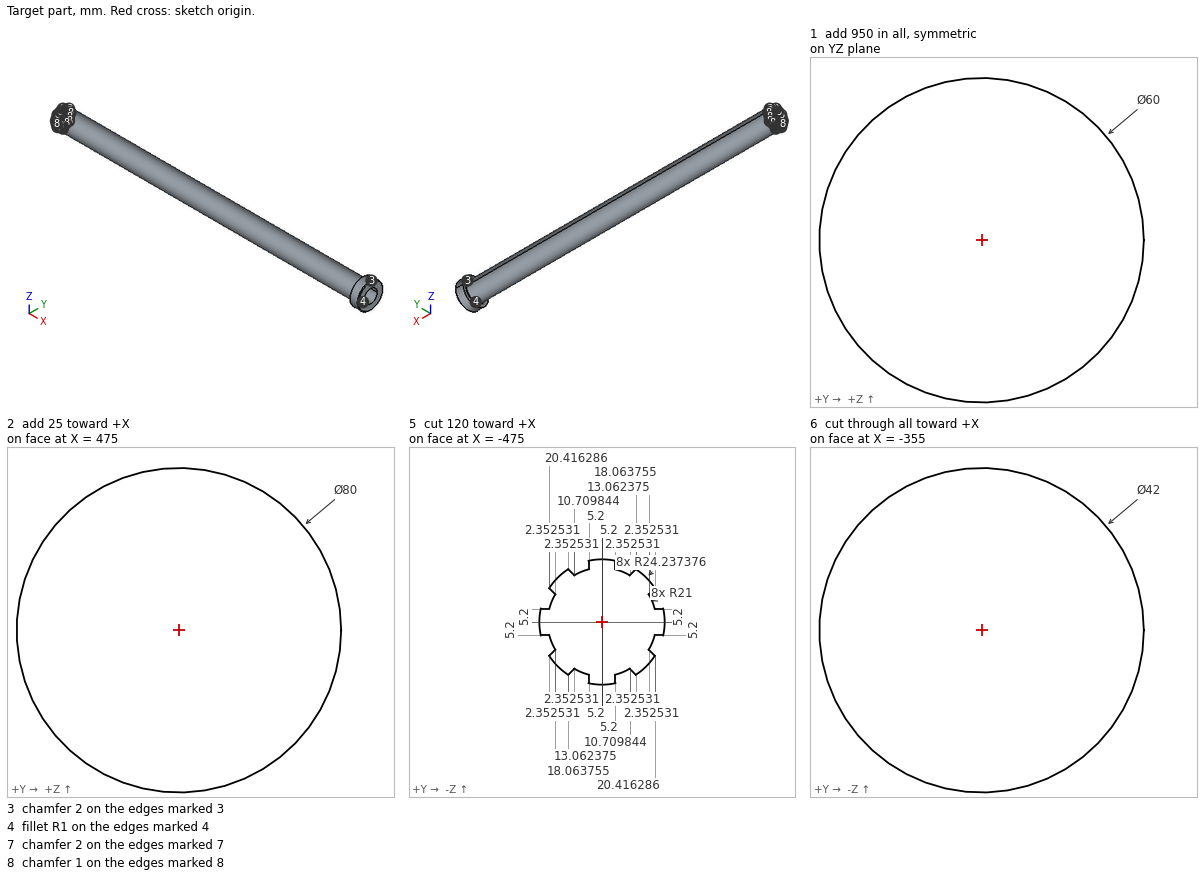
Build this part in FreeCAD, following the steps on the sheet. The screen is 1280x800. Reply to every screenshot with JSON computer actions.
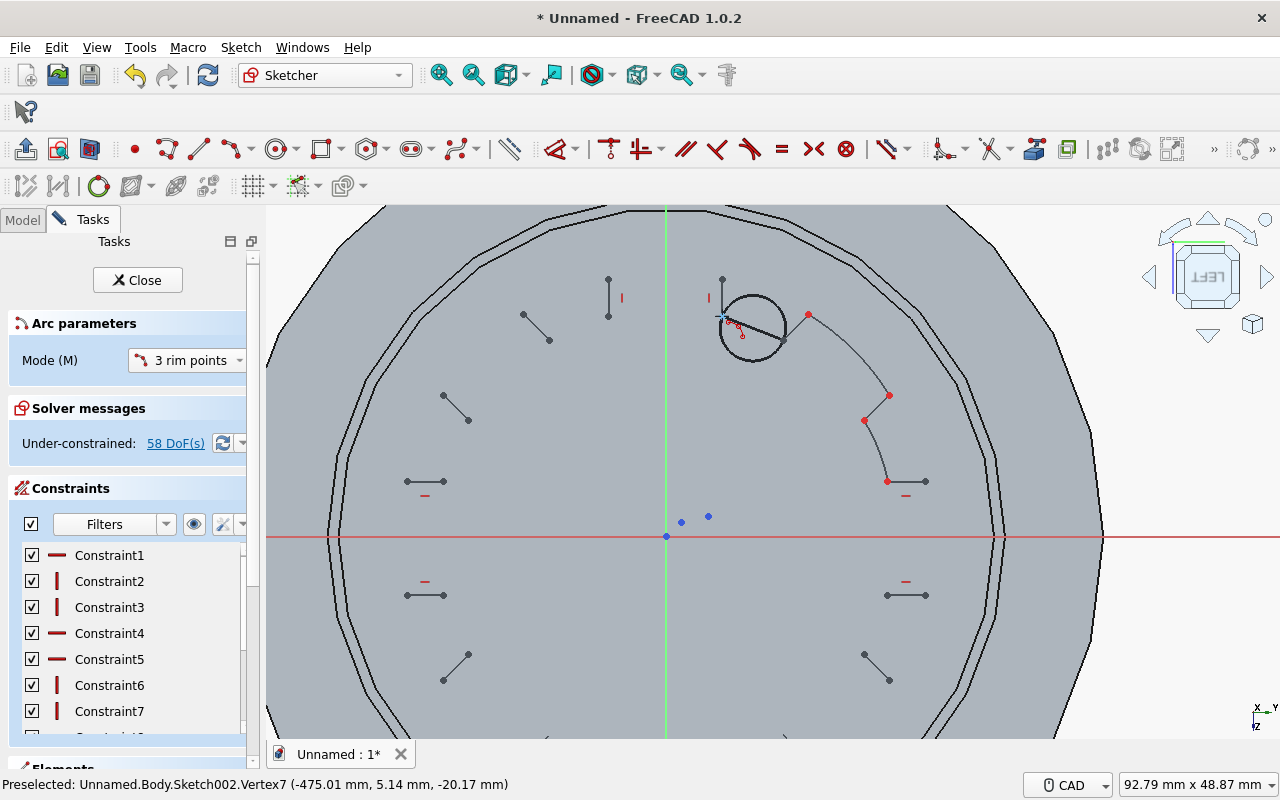
{"action": "scroll", "coordinate": [754, 325], "scroll_direction": "up", "scroll_amount": 10}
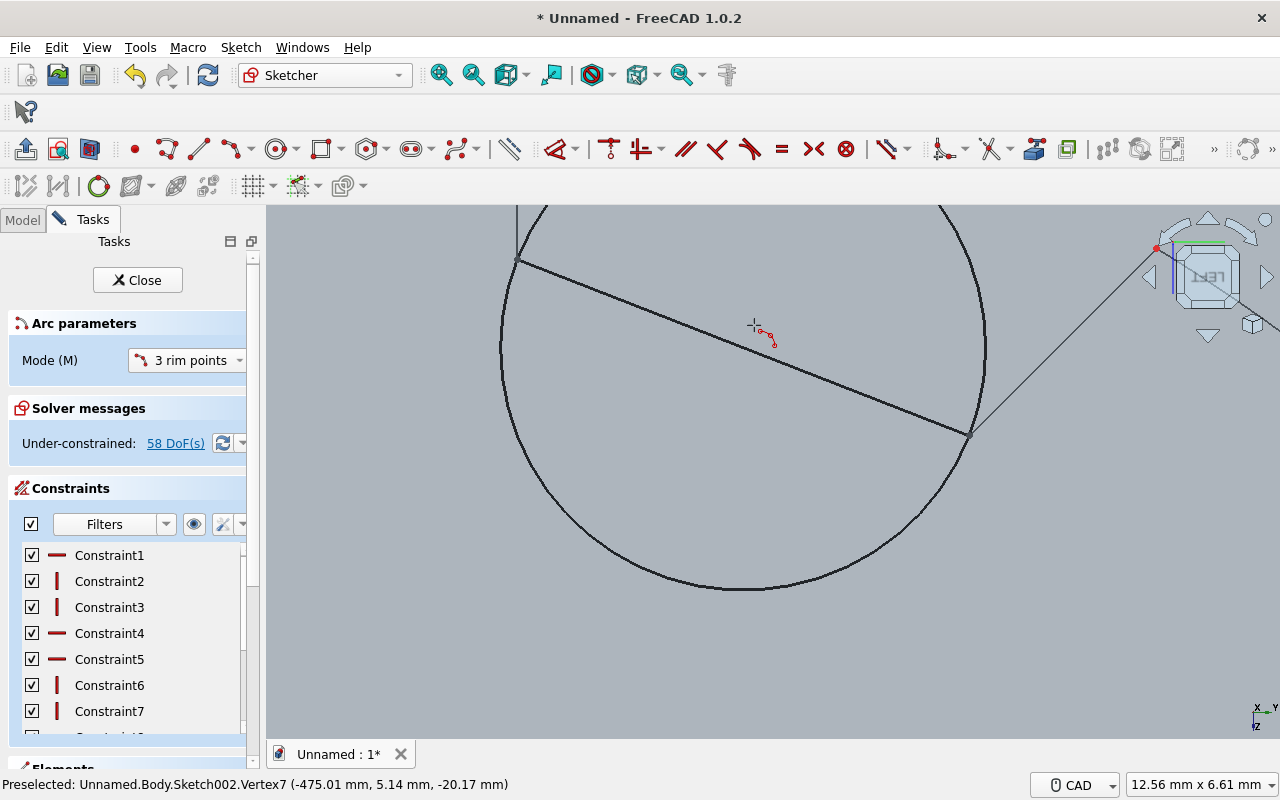
{"action": "left_click", "coordinate": [751, 322]}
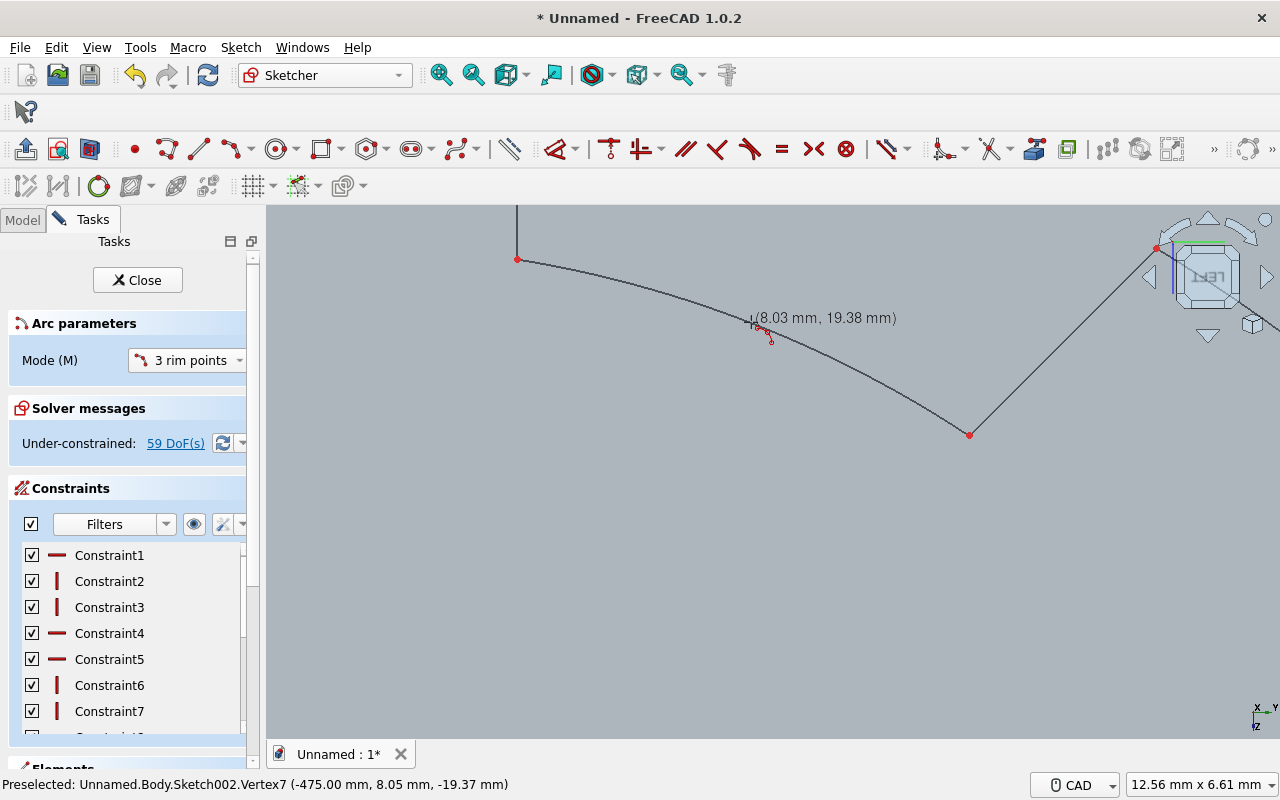
{"action": "scroll", "coordinate": [765, 331], "scroll_direction": "down", "scroll_amount": 12}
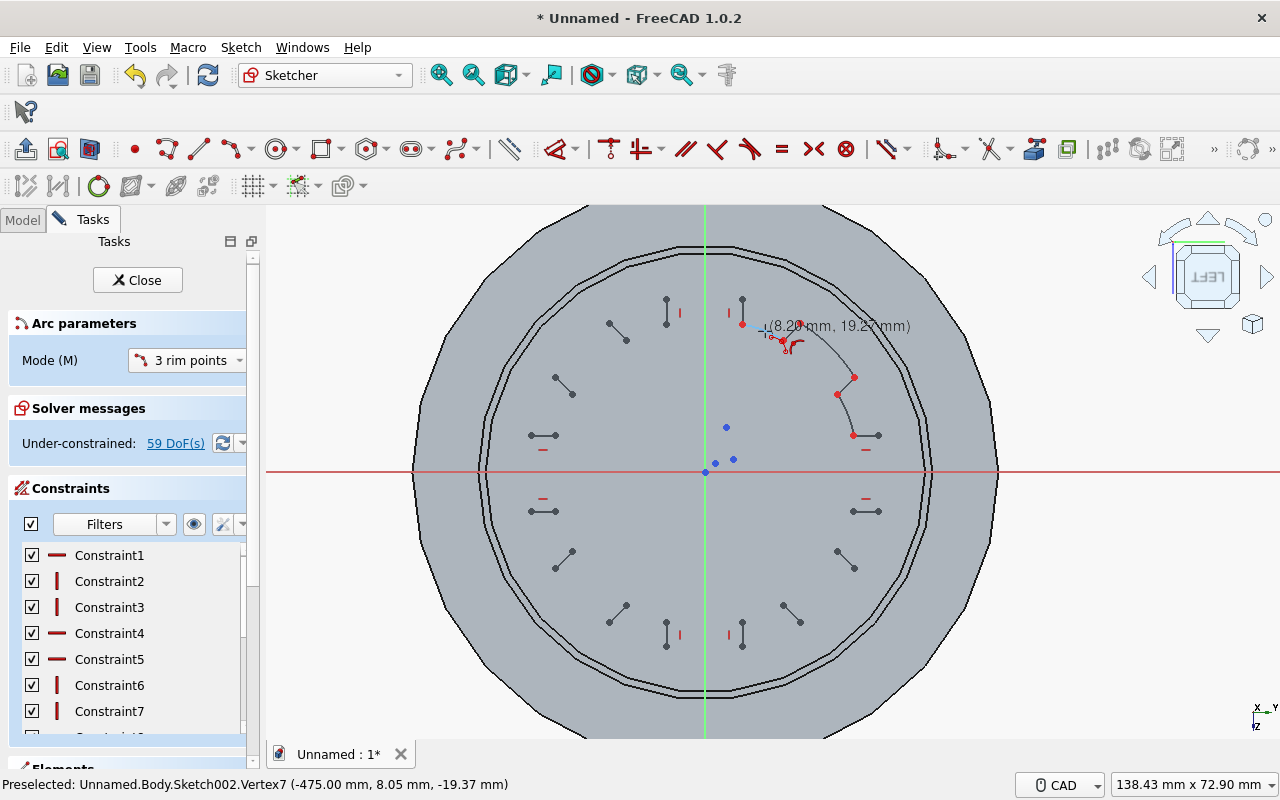
{"action": "scroll", "coordinate": [743, 299], "scroll_direction": "up", "scroll_amount": 2}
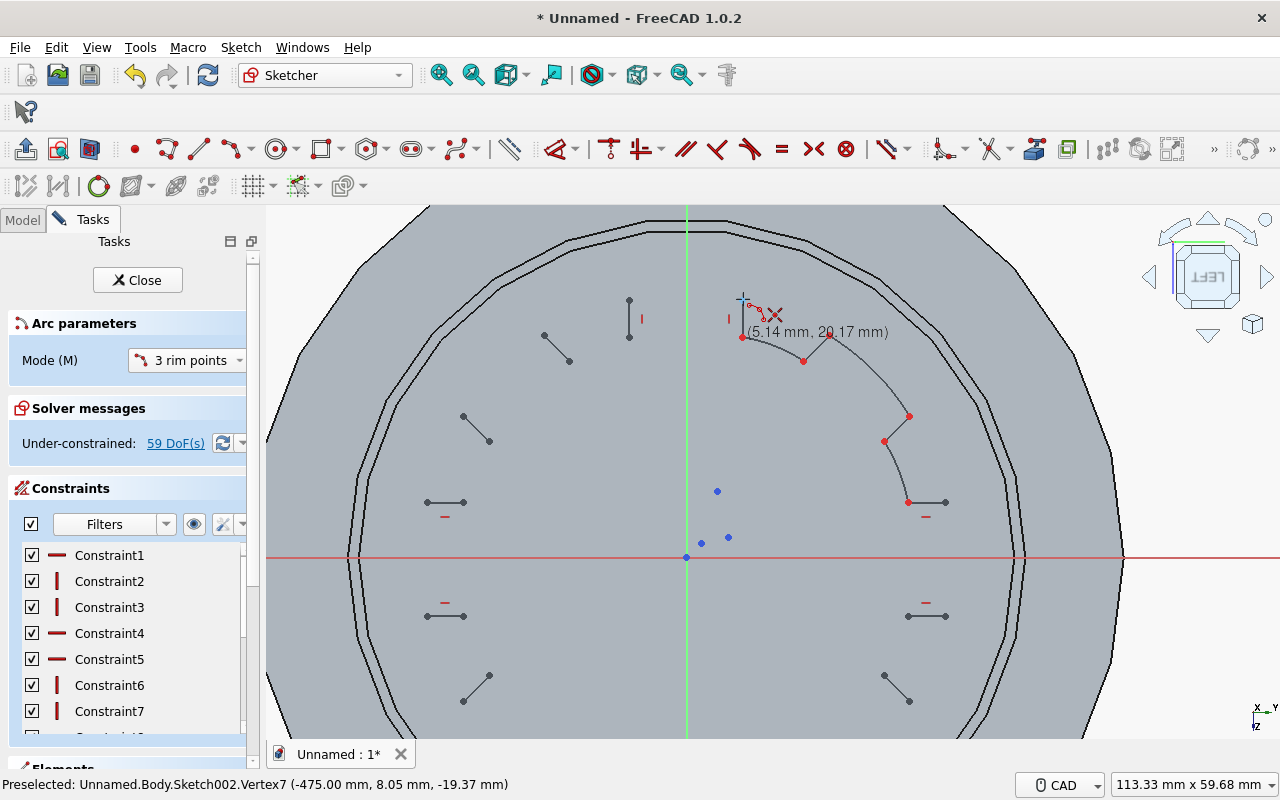
{"action": "left_click", "coordinate": [743, 300]}
{"action": "left_click", "coordinate": [629, 300]}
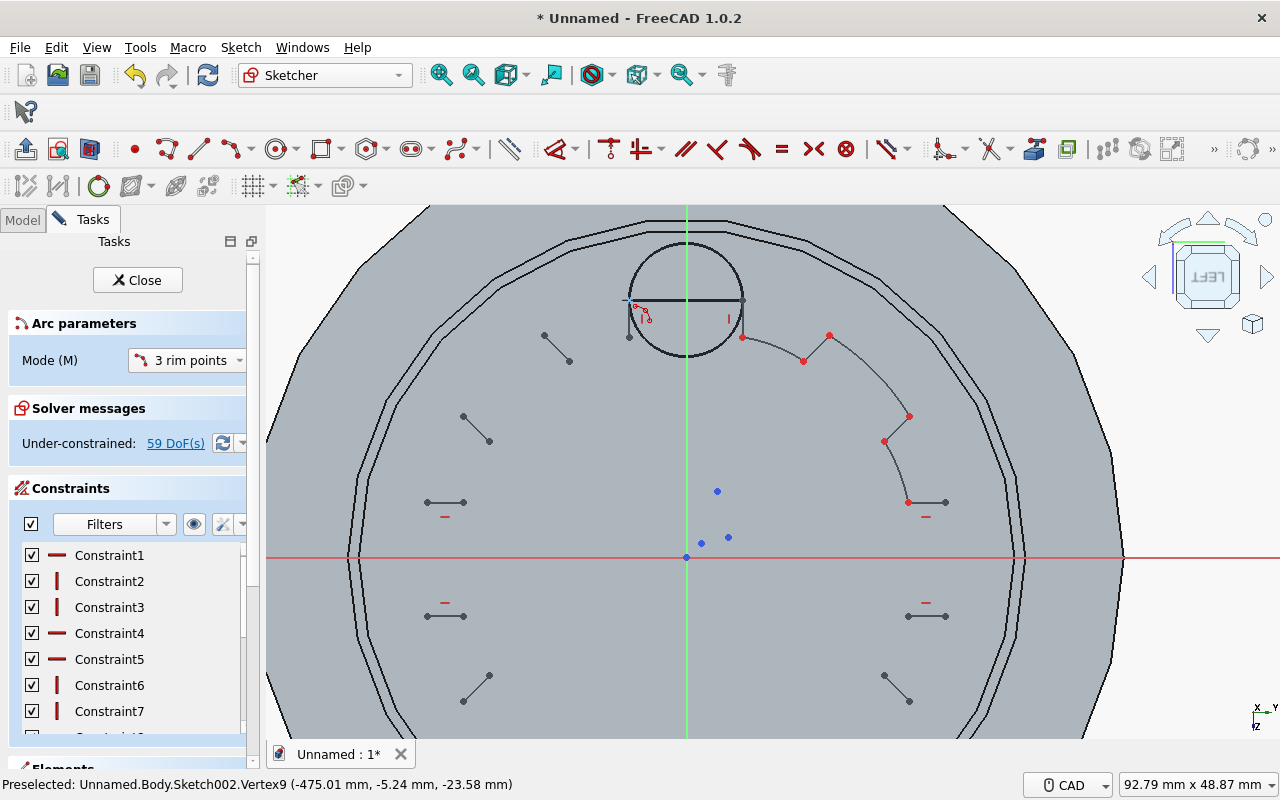
{"action": "scroll", "coordinate": [698, 293], "scroll_direction": "up", "scroll_amount": 5}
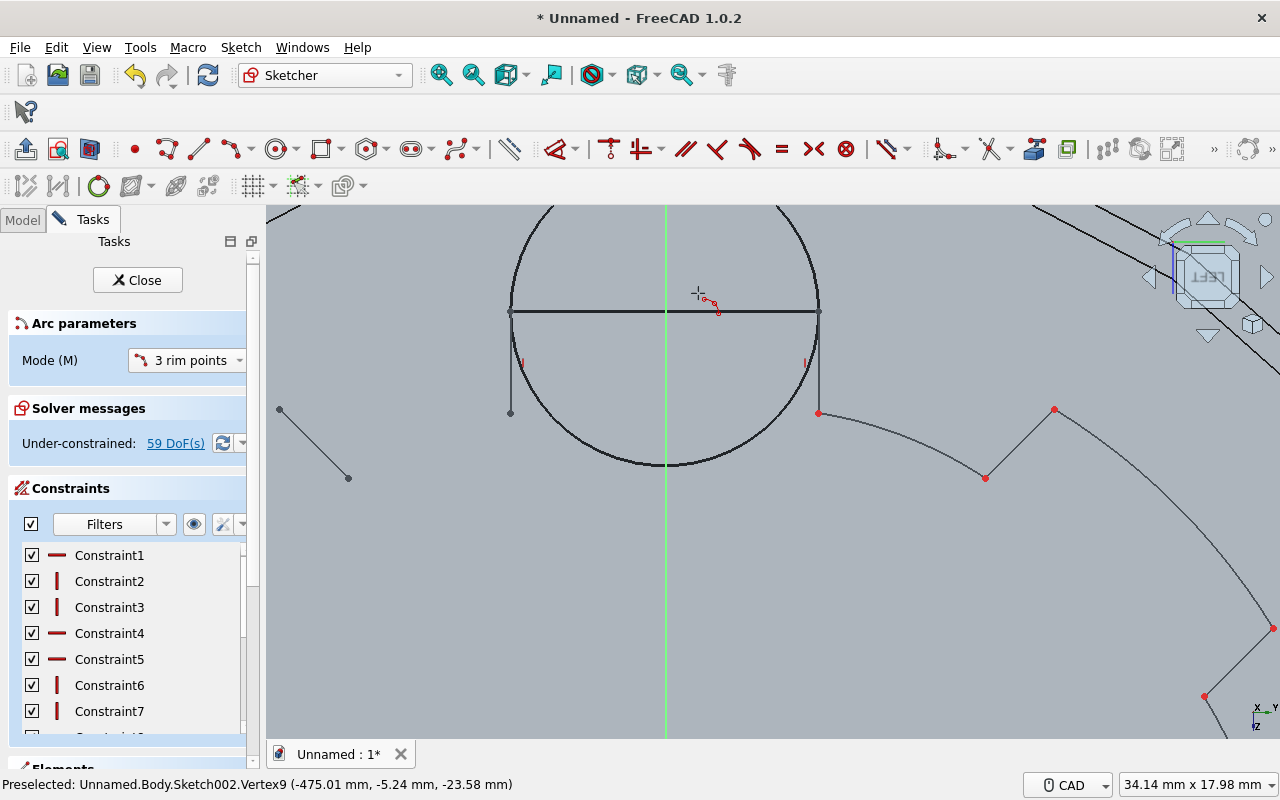
{"action": "left_click", "coordinate": [697, 293]}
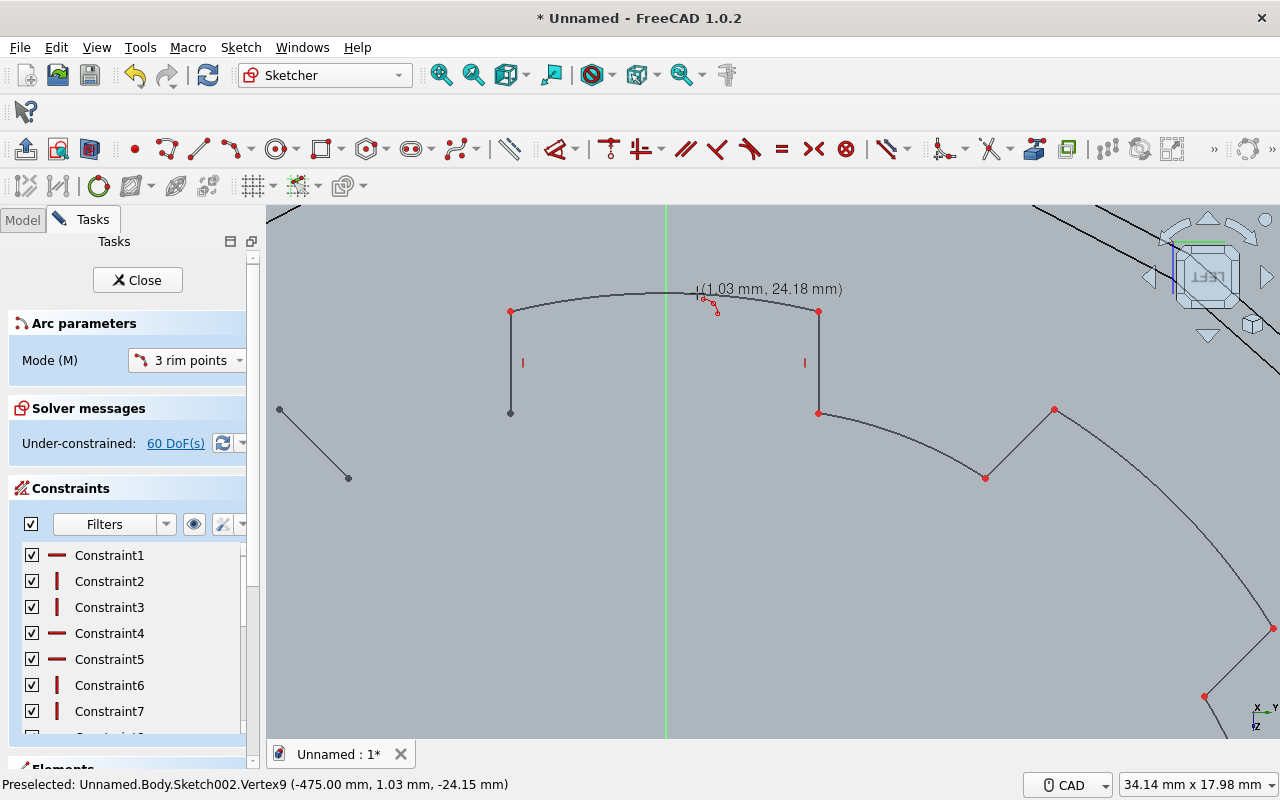
{"action": "scroll", "coordinate": [717, 295], "scroll_direction": "down", "scroll_amount": 7}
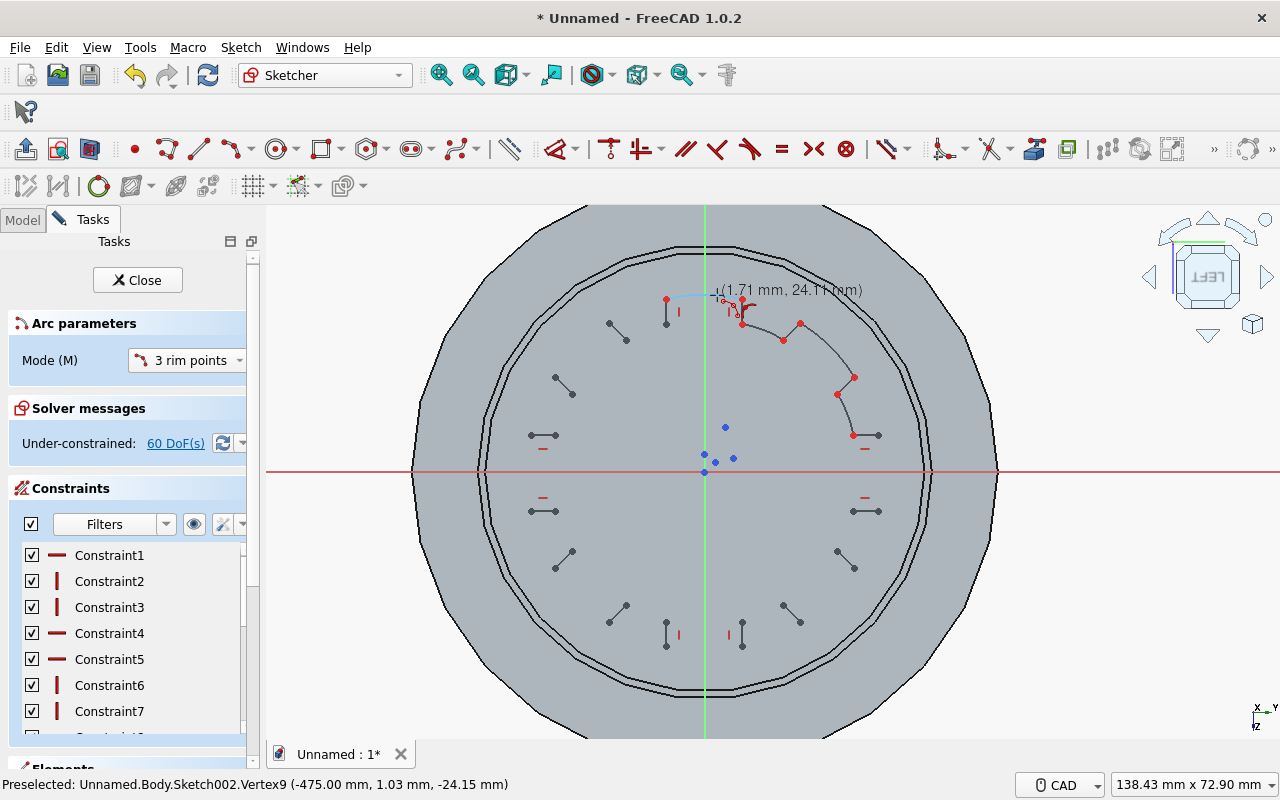
{"action": "scroll", "coordinate": [667, 323], "scroll_direction": "up", "scroll_amount": 2}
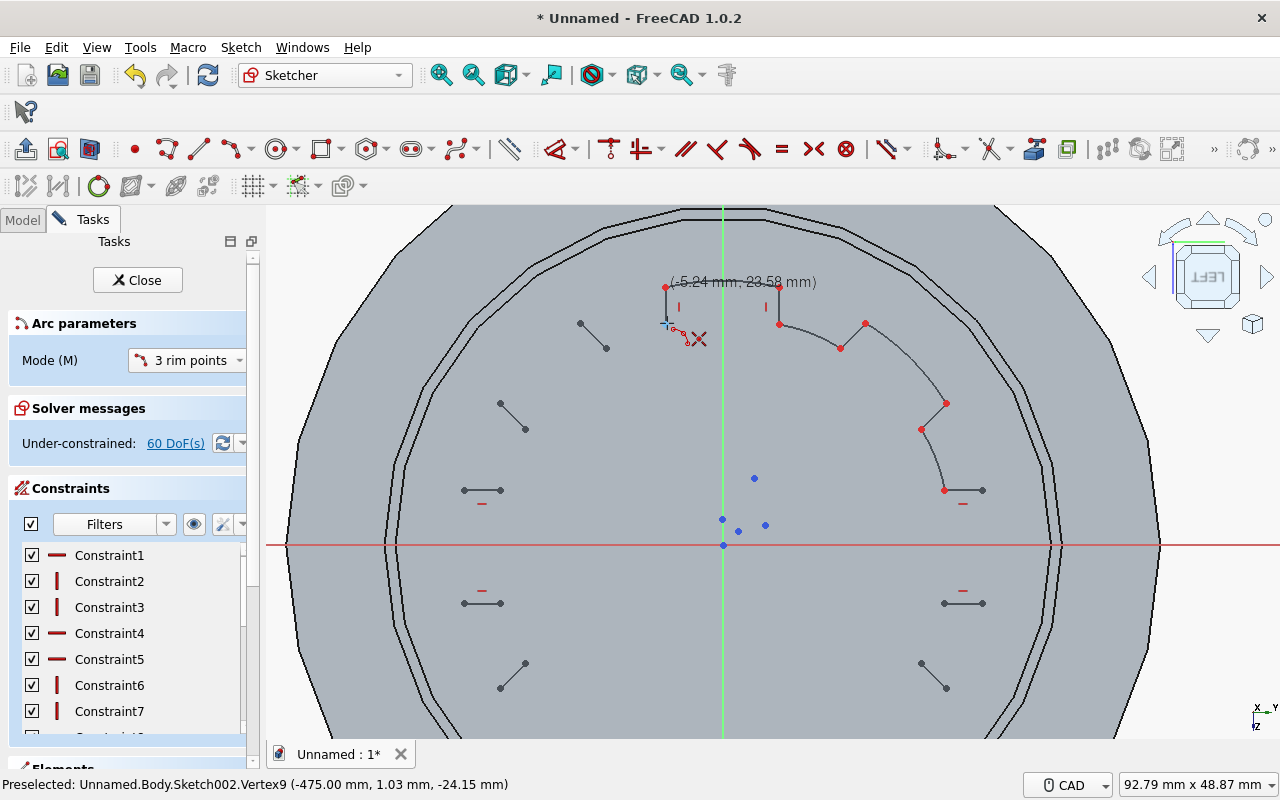
{"action": "left_click", "coordinate": [666, 325]}
{"action": "left_click", "coordinate": [606, 349]}